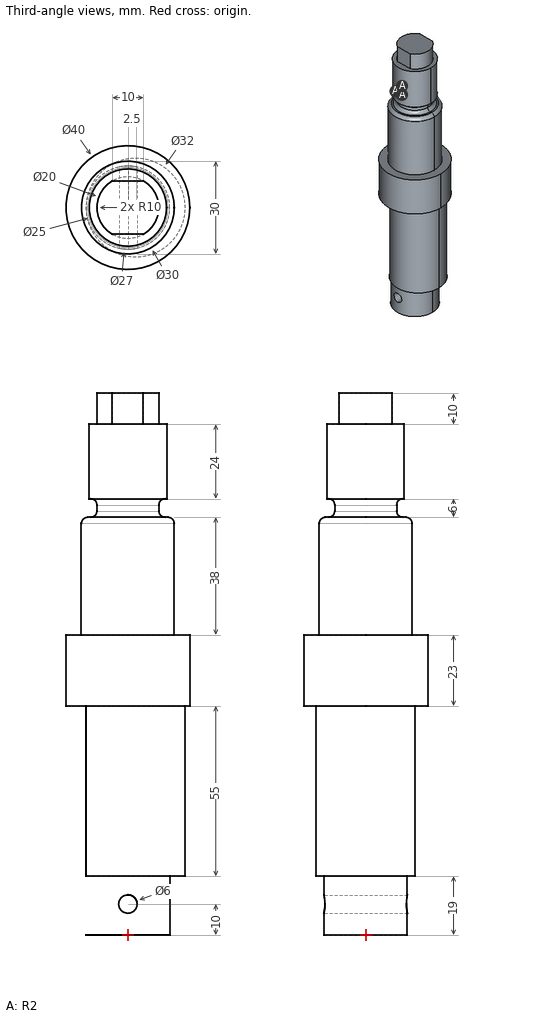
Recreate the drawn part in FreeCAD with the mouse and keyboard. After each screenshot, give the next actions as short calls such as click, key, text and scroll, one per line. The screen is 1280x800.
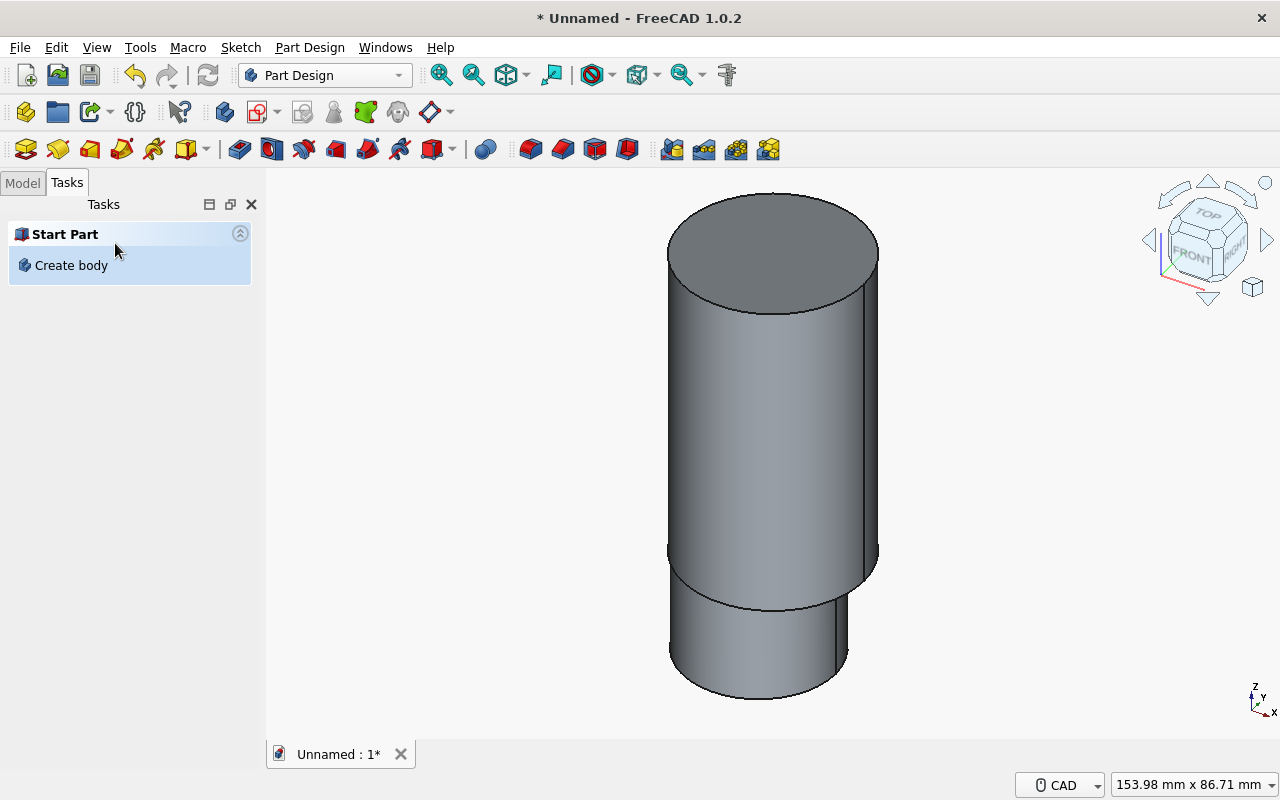
click(773, 253)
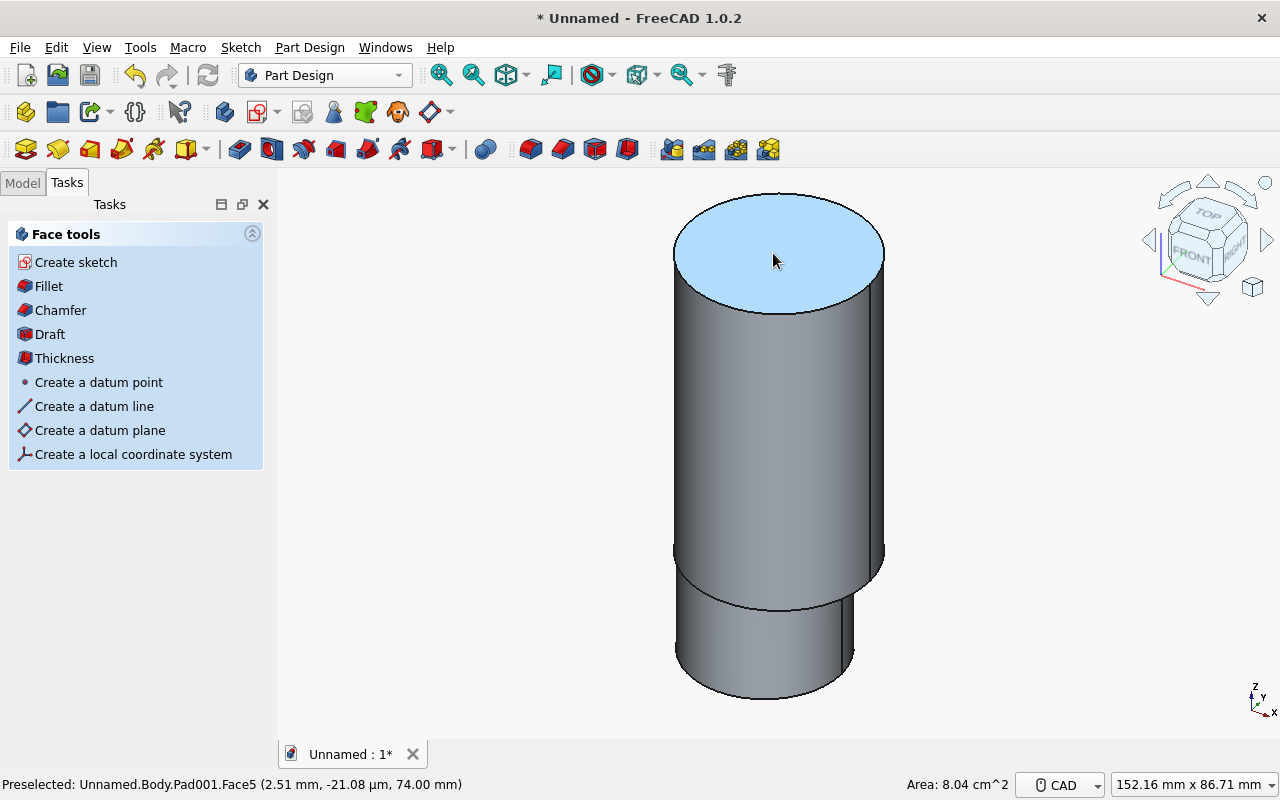
click(258, 112)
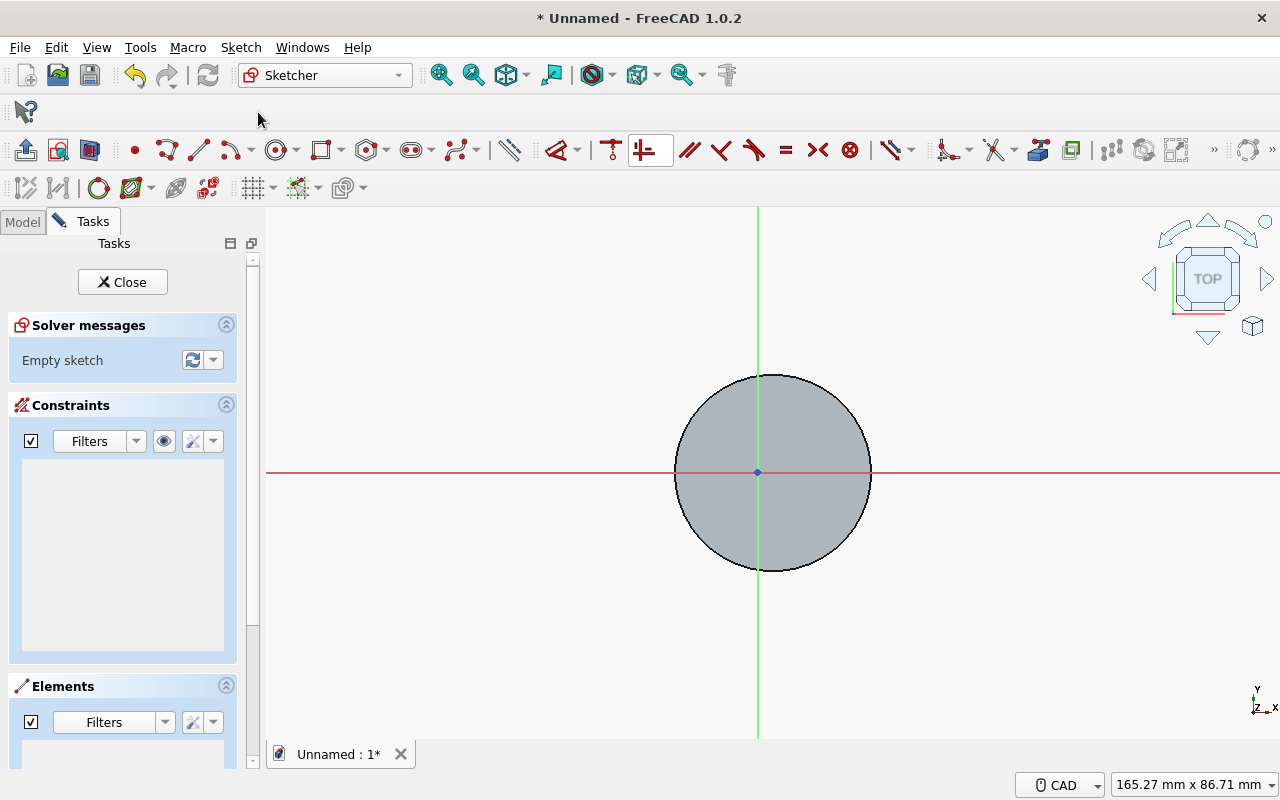
scroll(866, 473, up, 2)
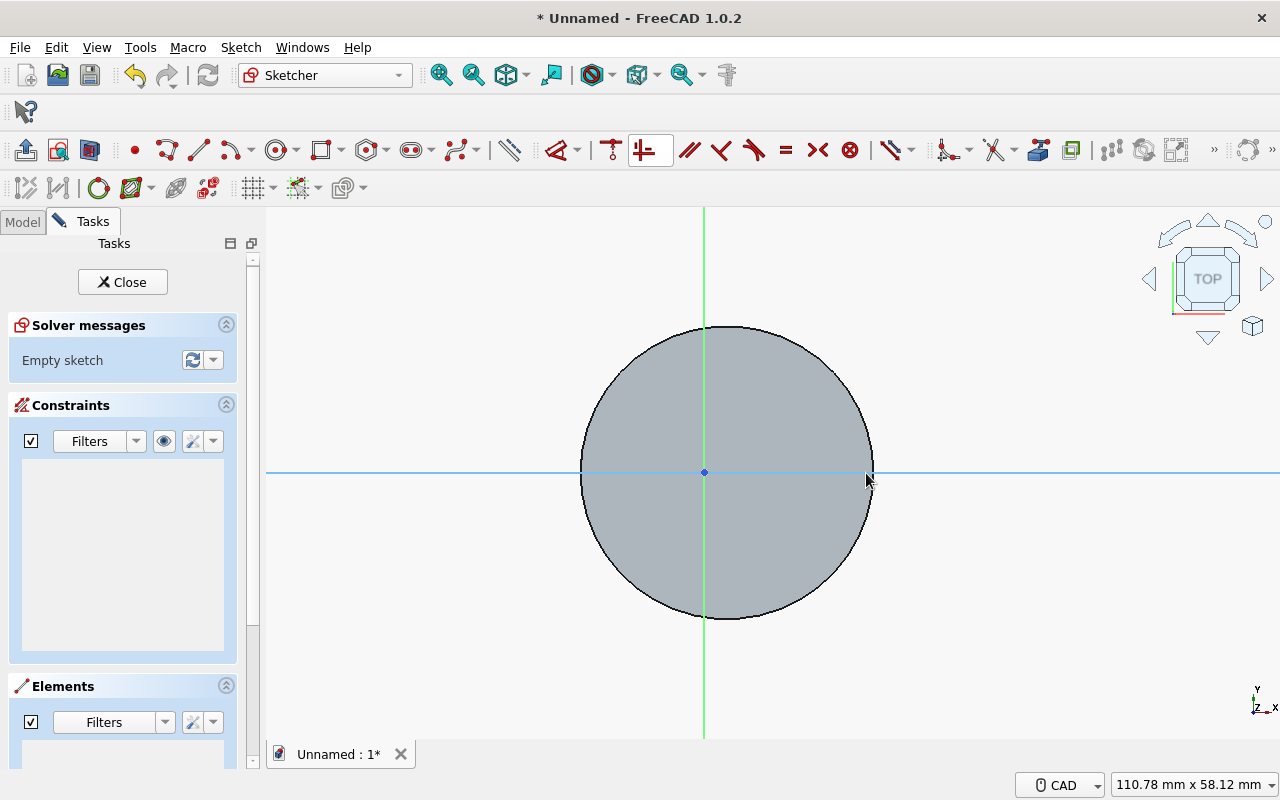
key(g)
key(c)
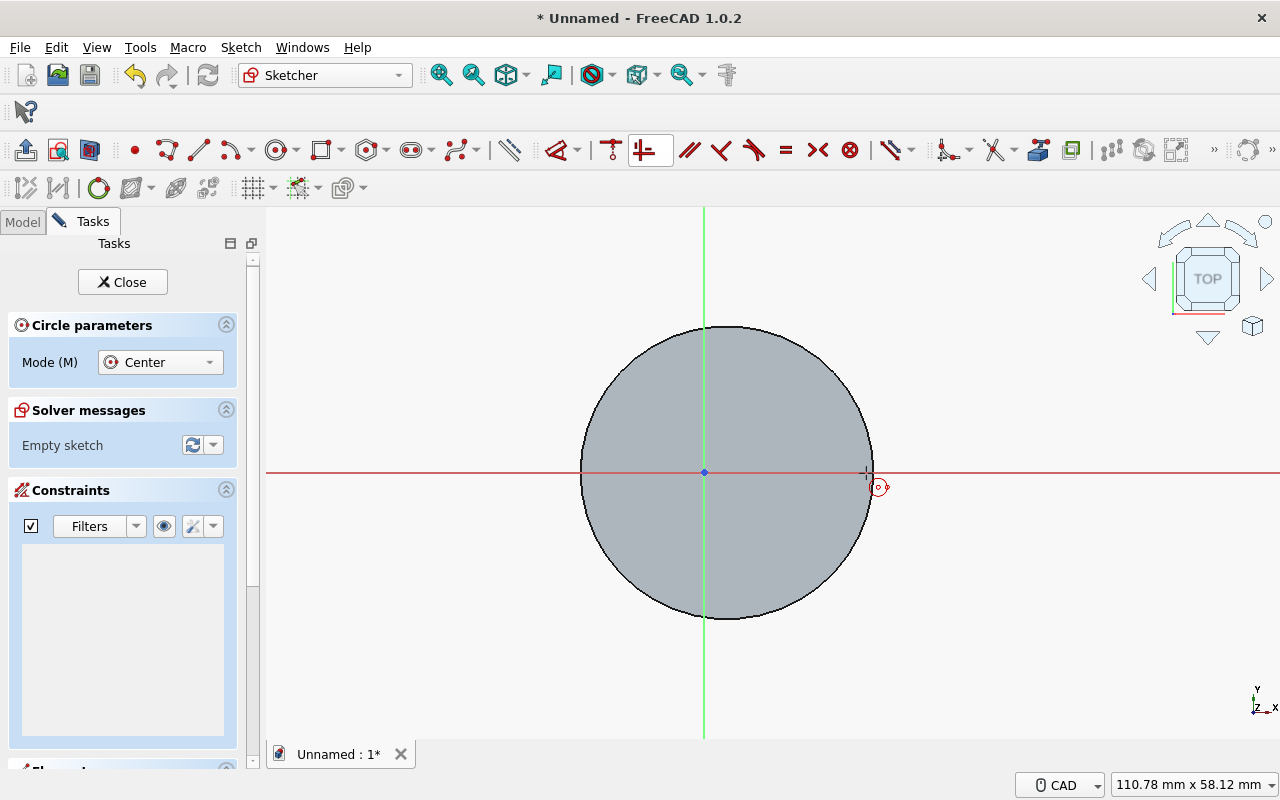
click(704, 473)
click(834, 343)
key(Escape)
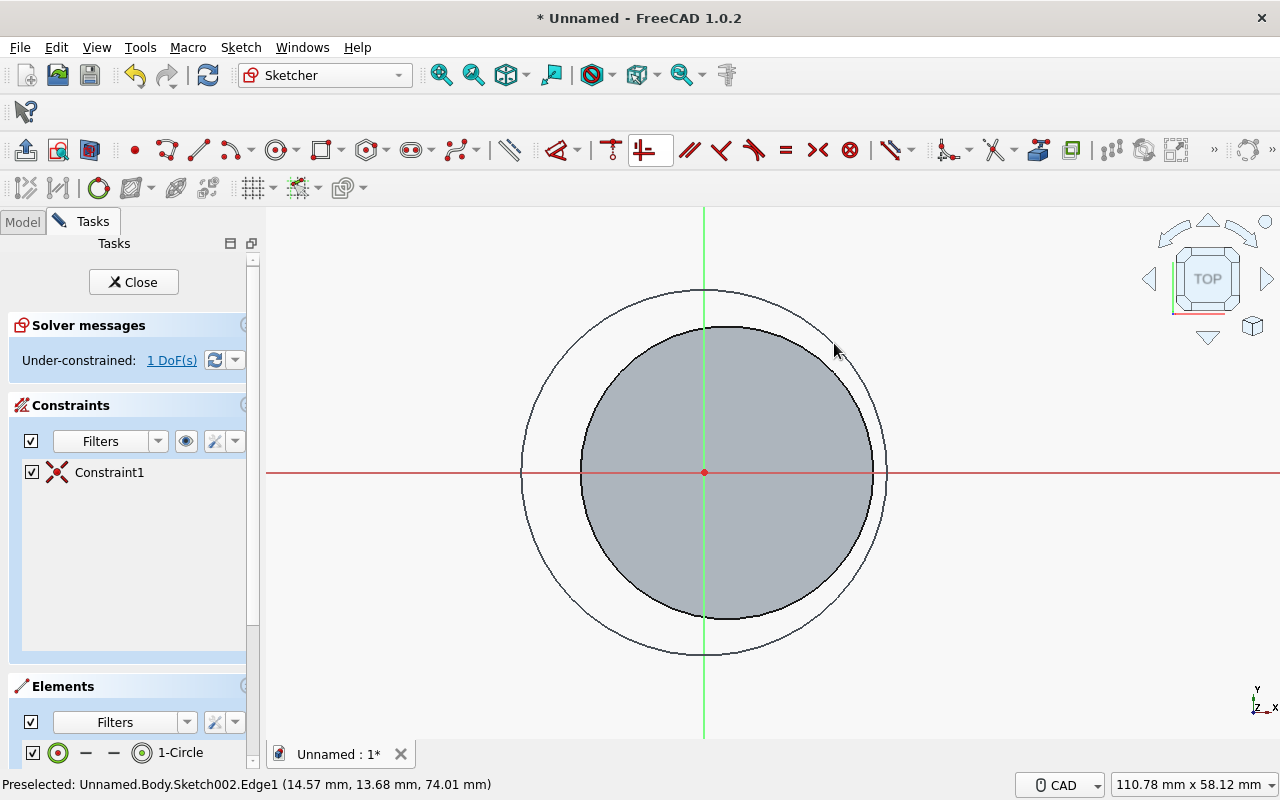
key(d)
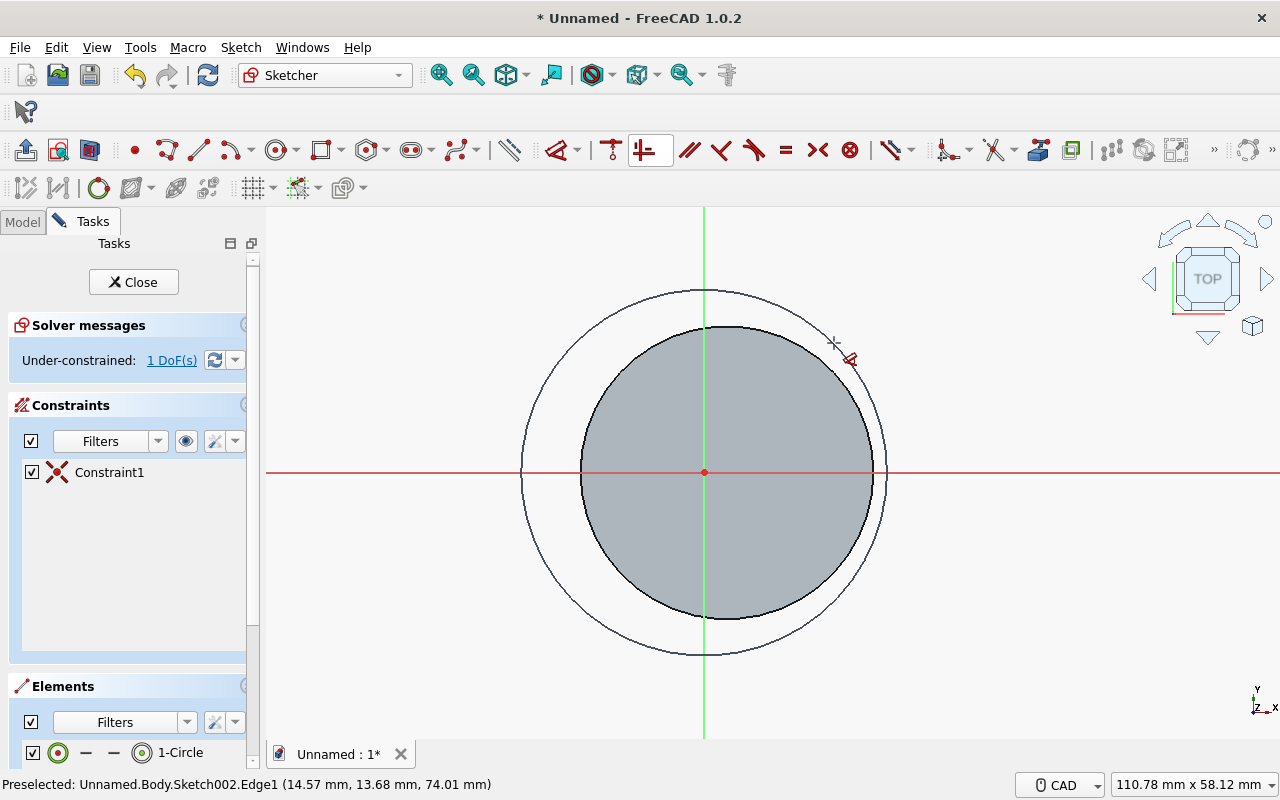
click(833, 343)
click(856, 320)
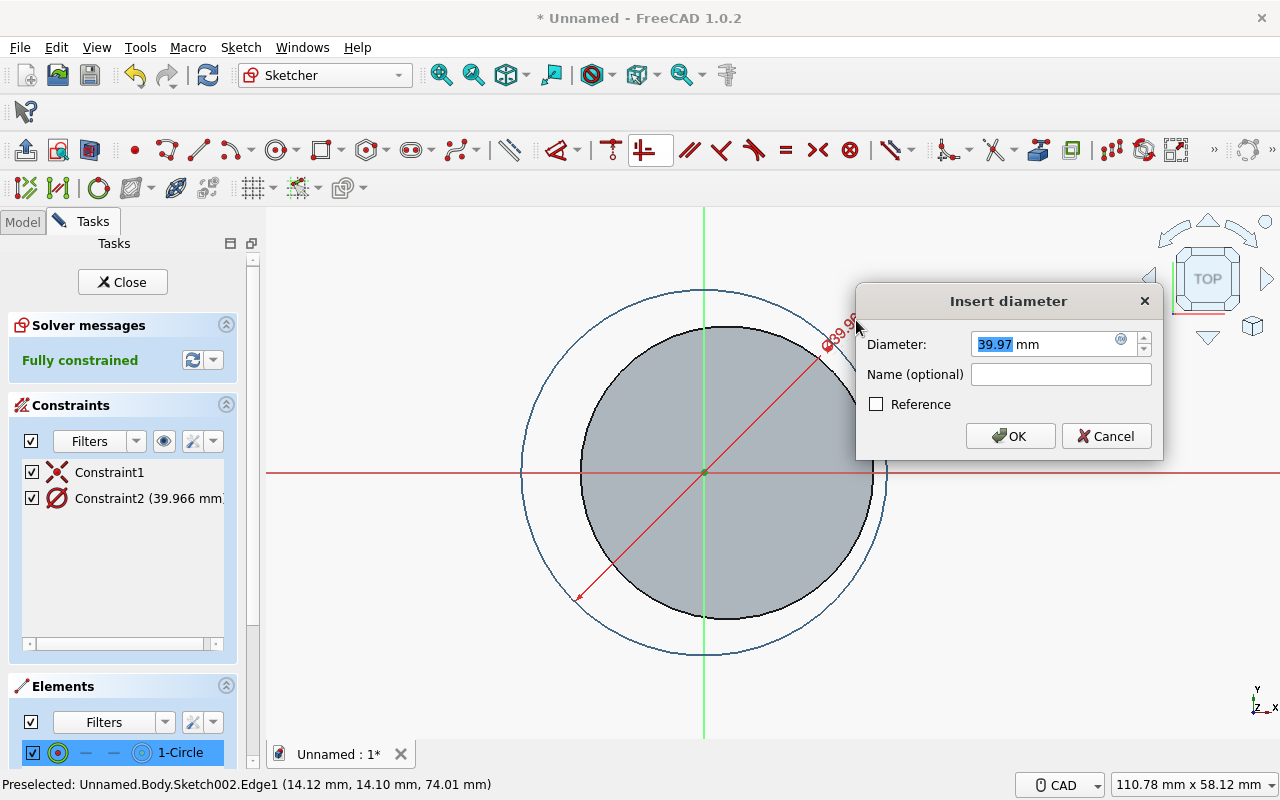
text(40)
key(Return)
key(Escape)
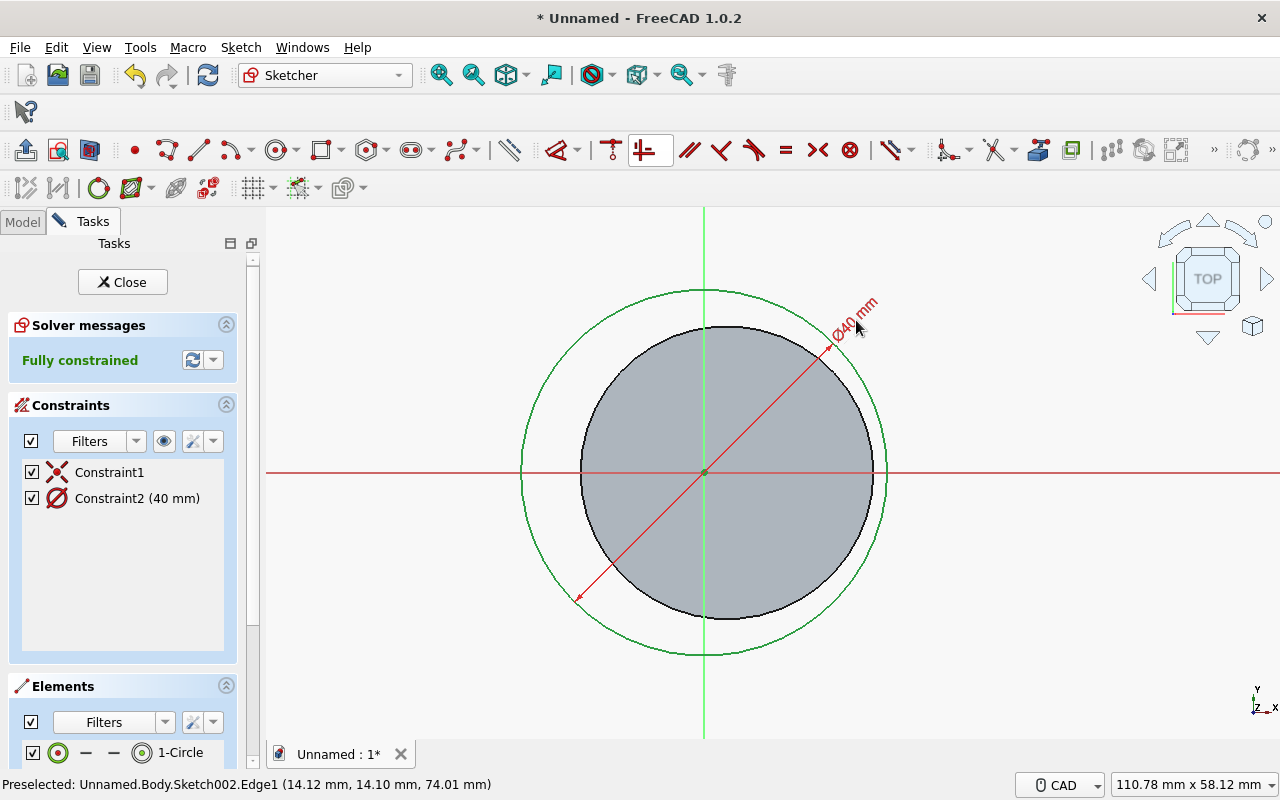
click(123, 282)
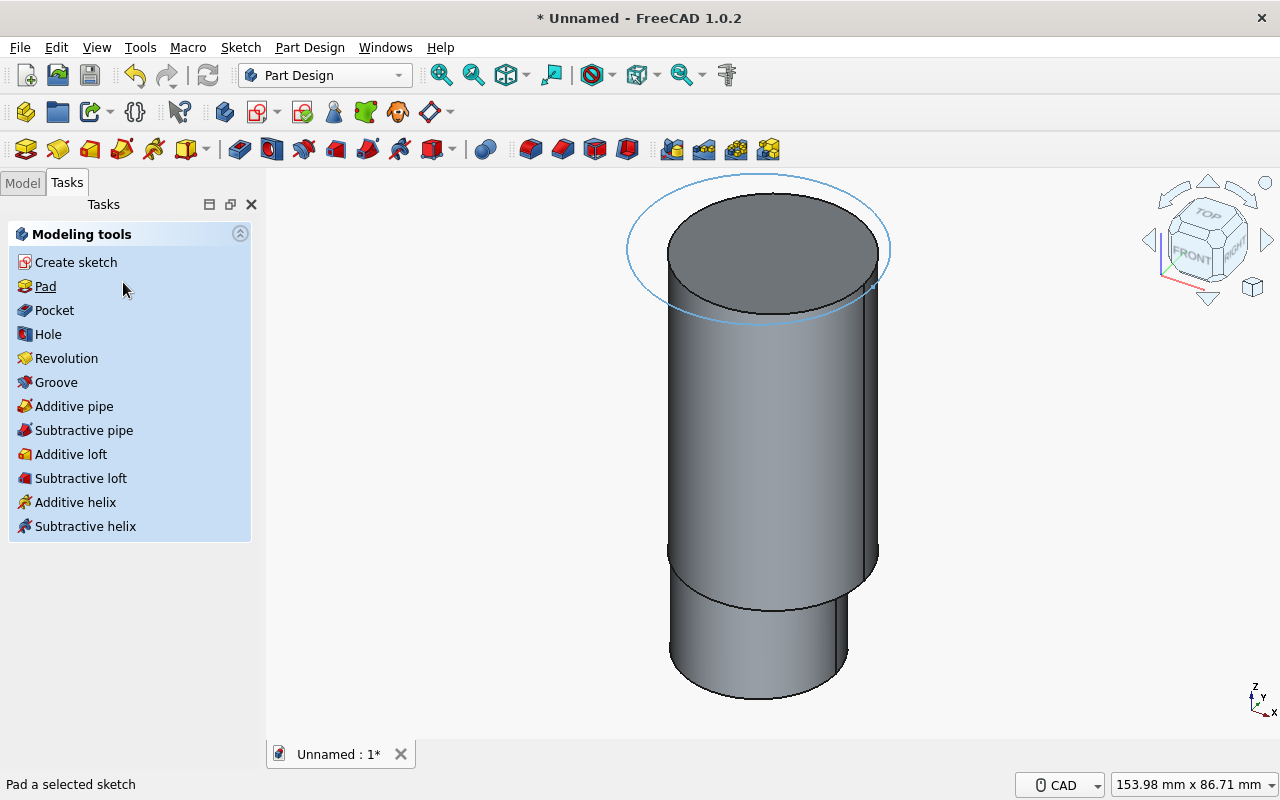
click(26, 150)